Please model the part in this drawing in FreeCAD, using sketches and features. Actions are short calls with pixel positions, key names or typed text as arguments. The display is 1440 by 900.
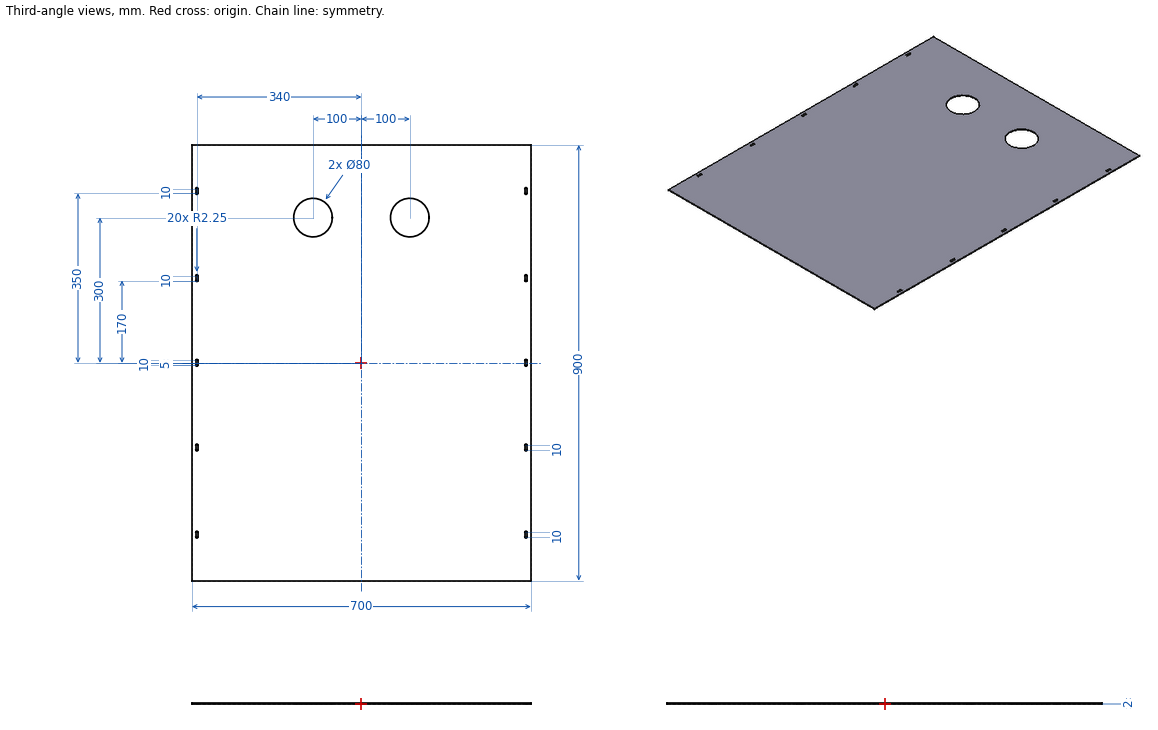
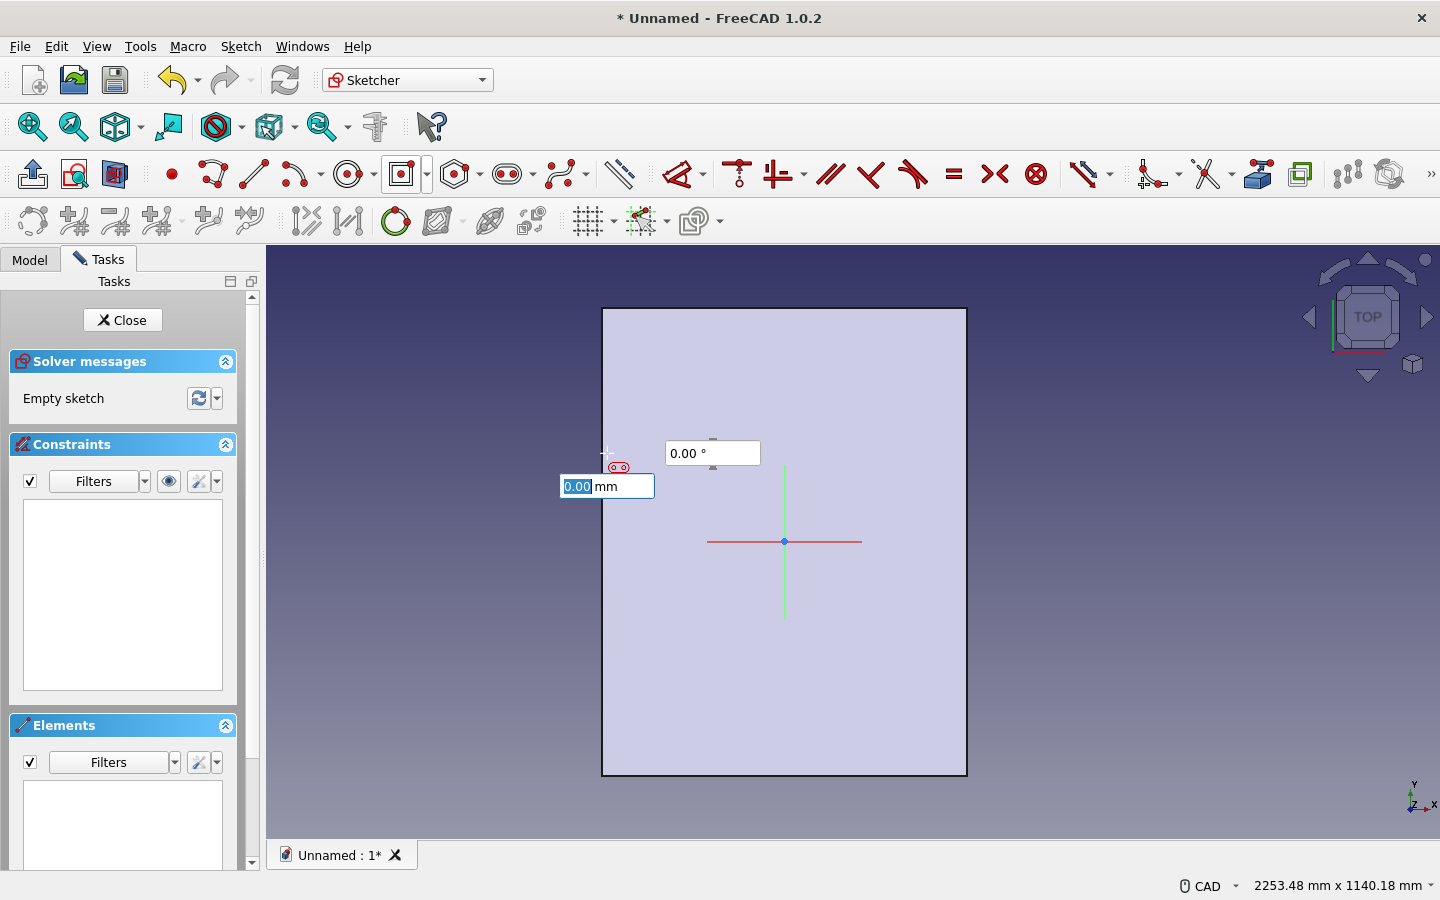
scroll(607, 448, up, 6)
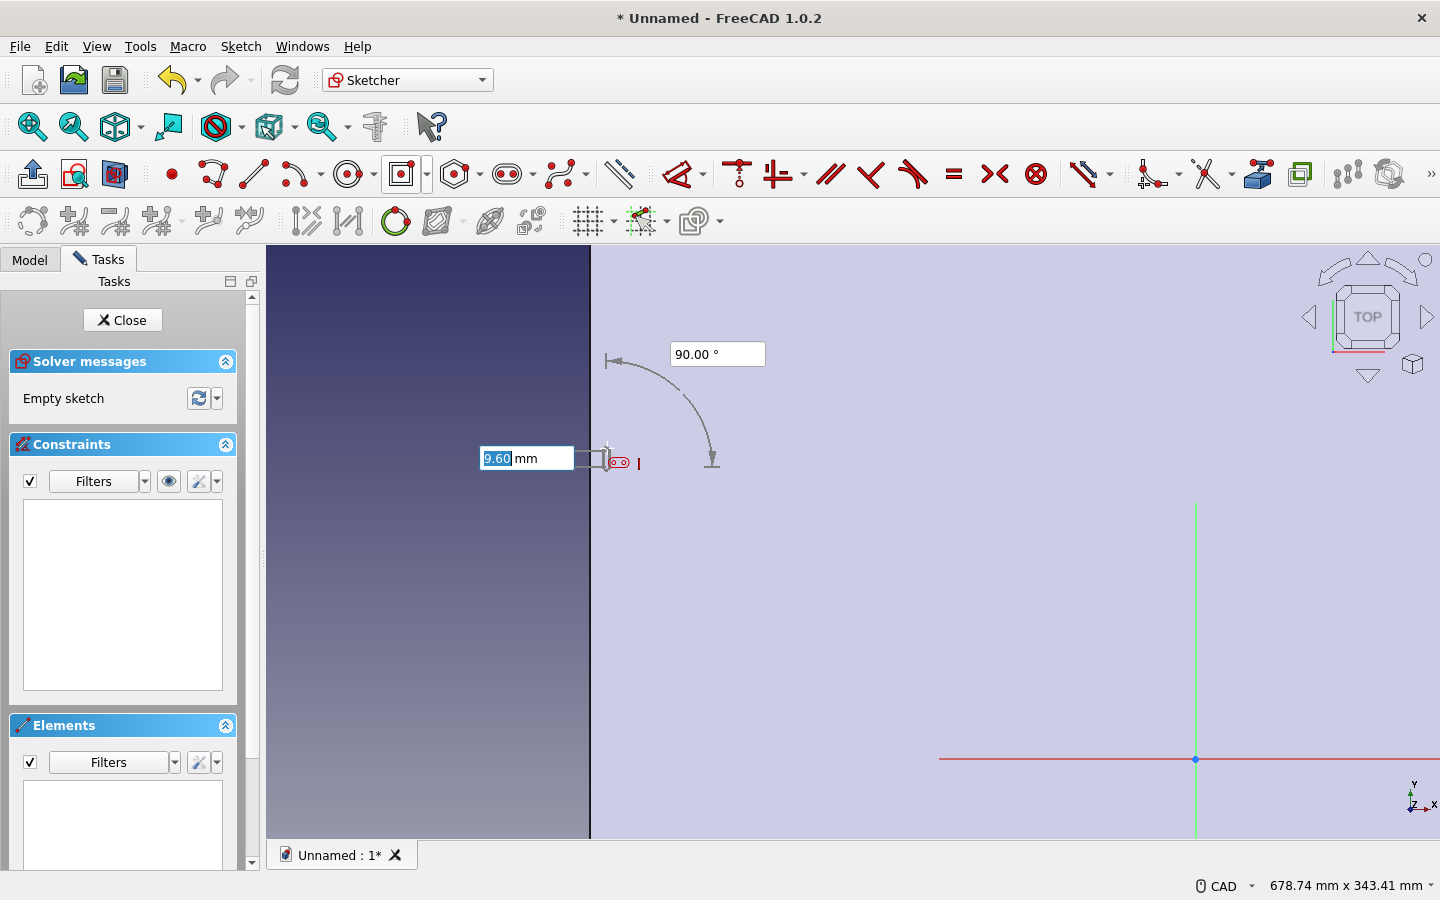
click(606, 448)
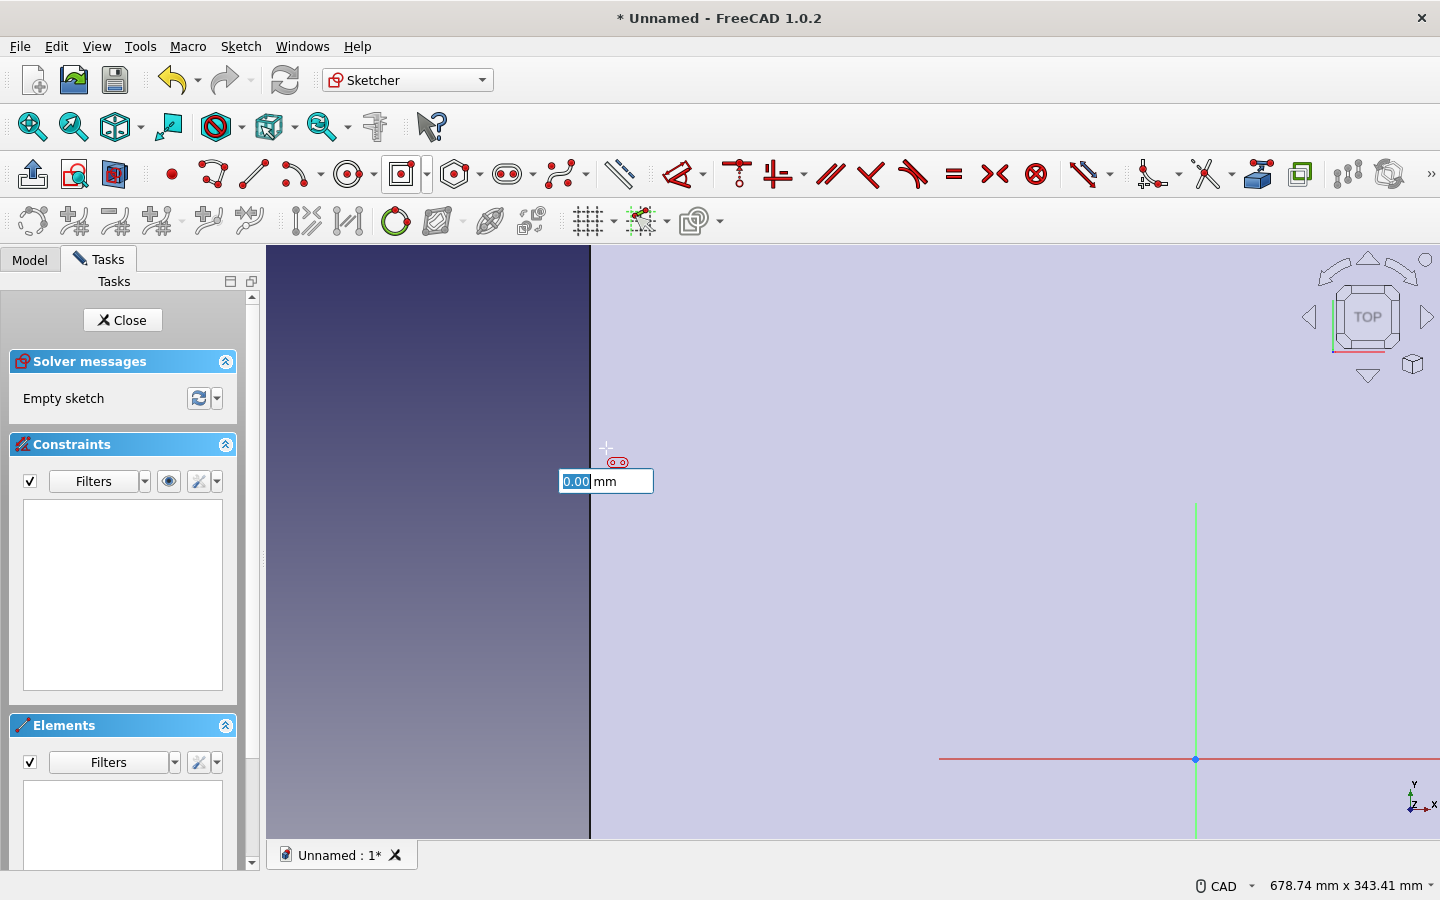
scroll(612, 457, up, 8)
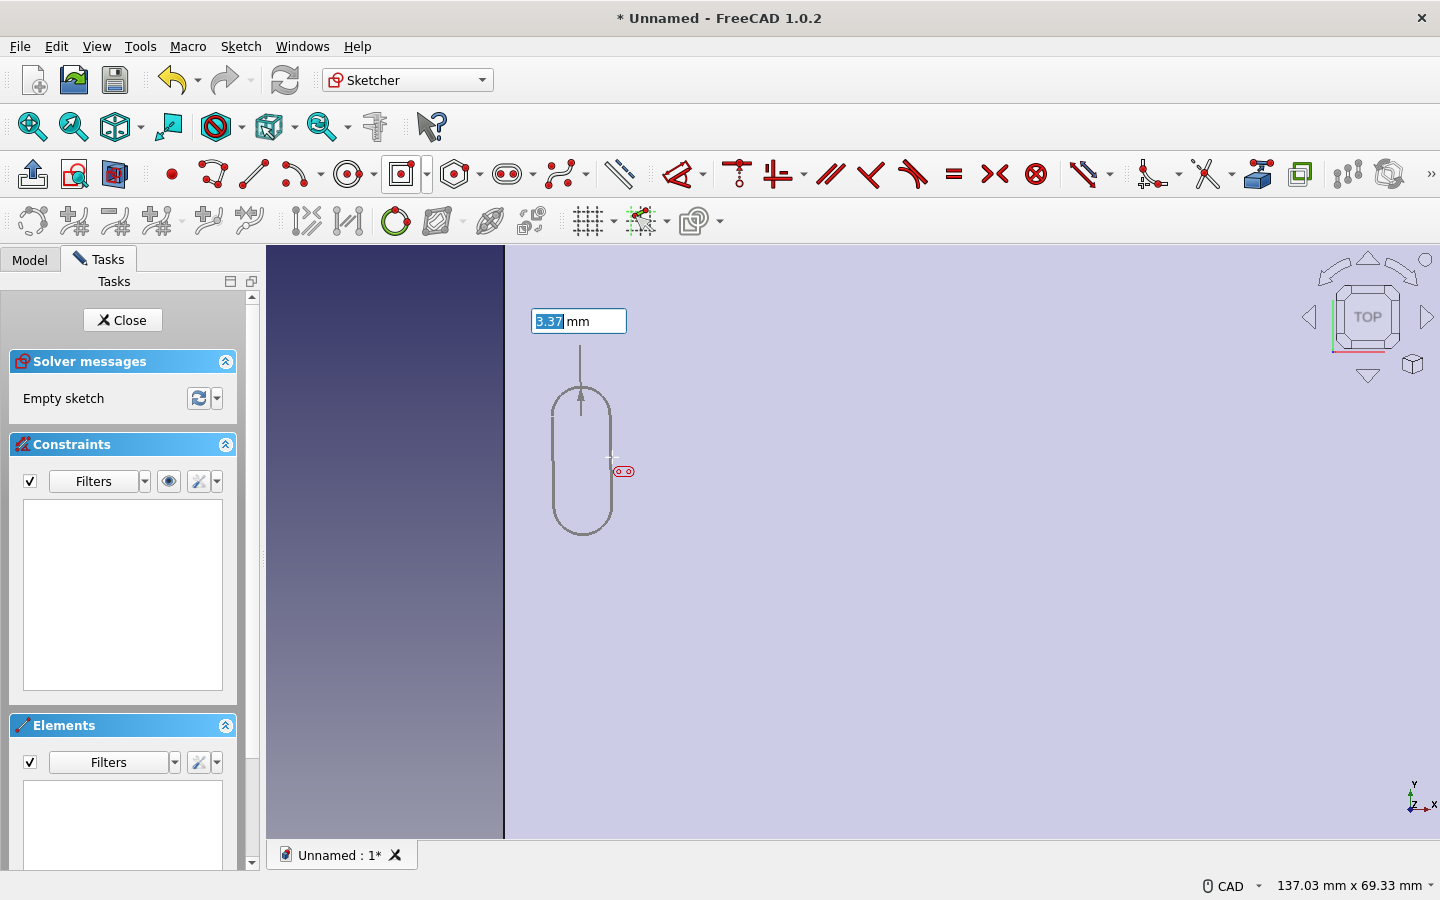
click(609, 454)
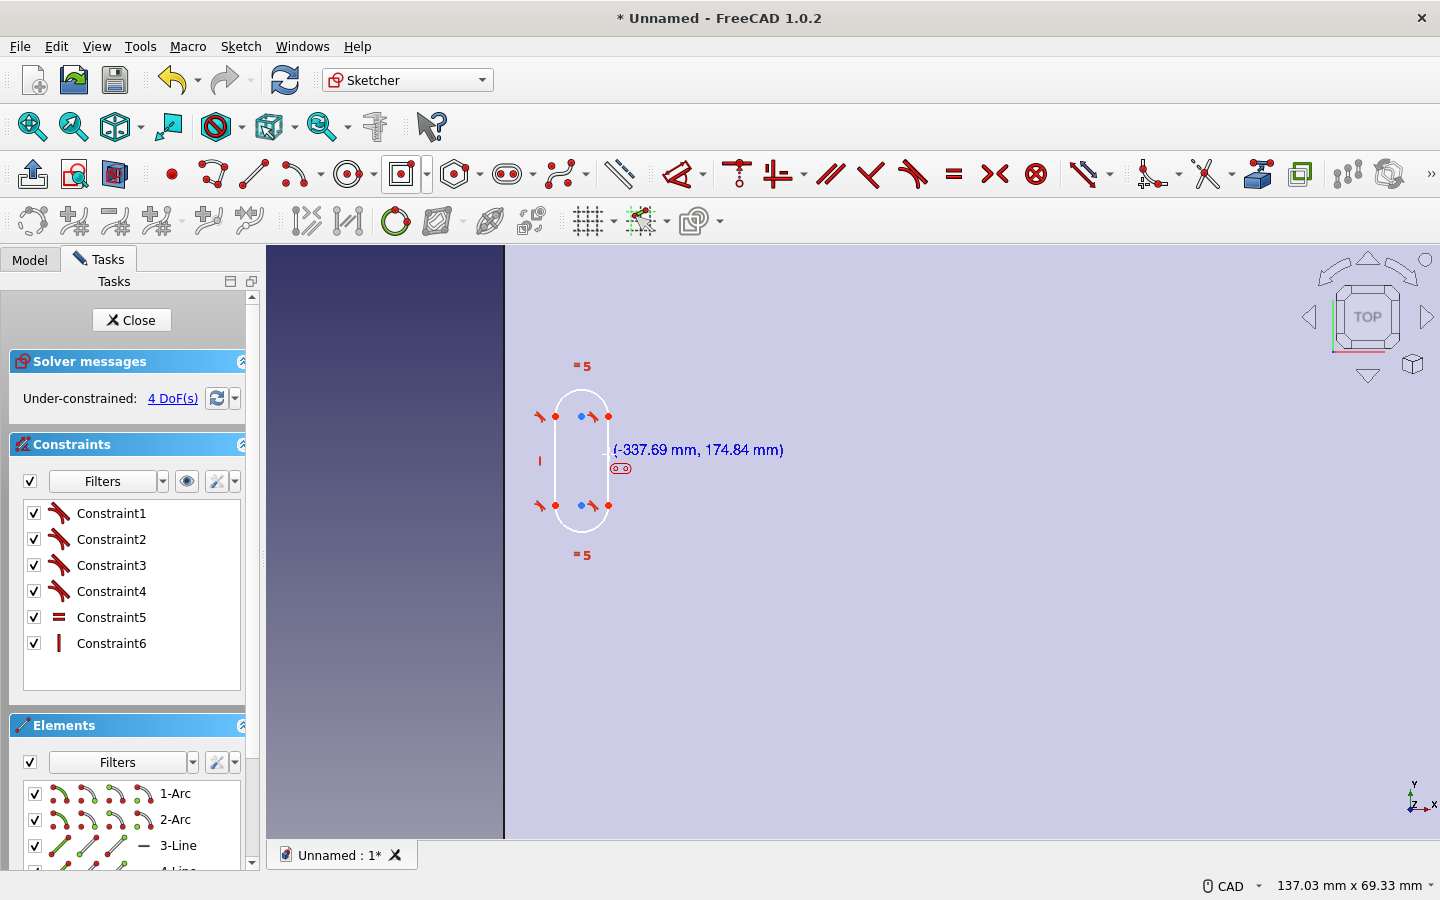
scroll(609, 451, down, 14)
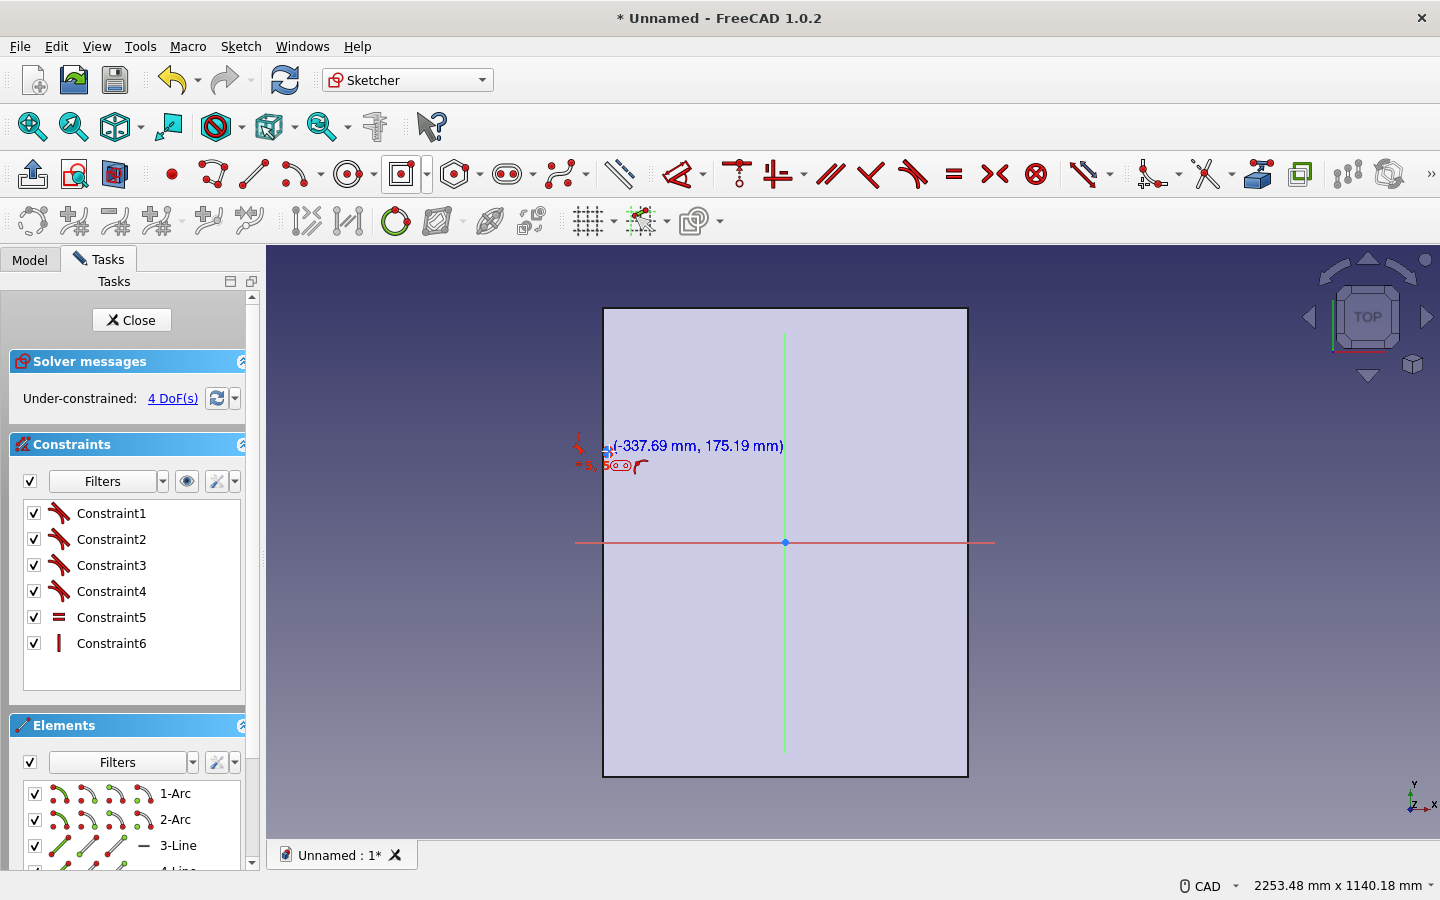
scroll(608, 545, up, 15)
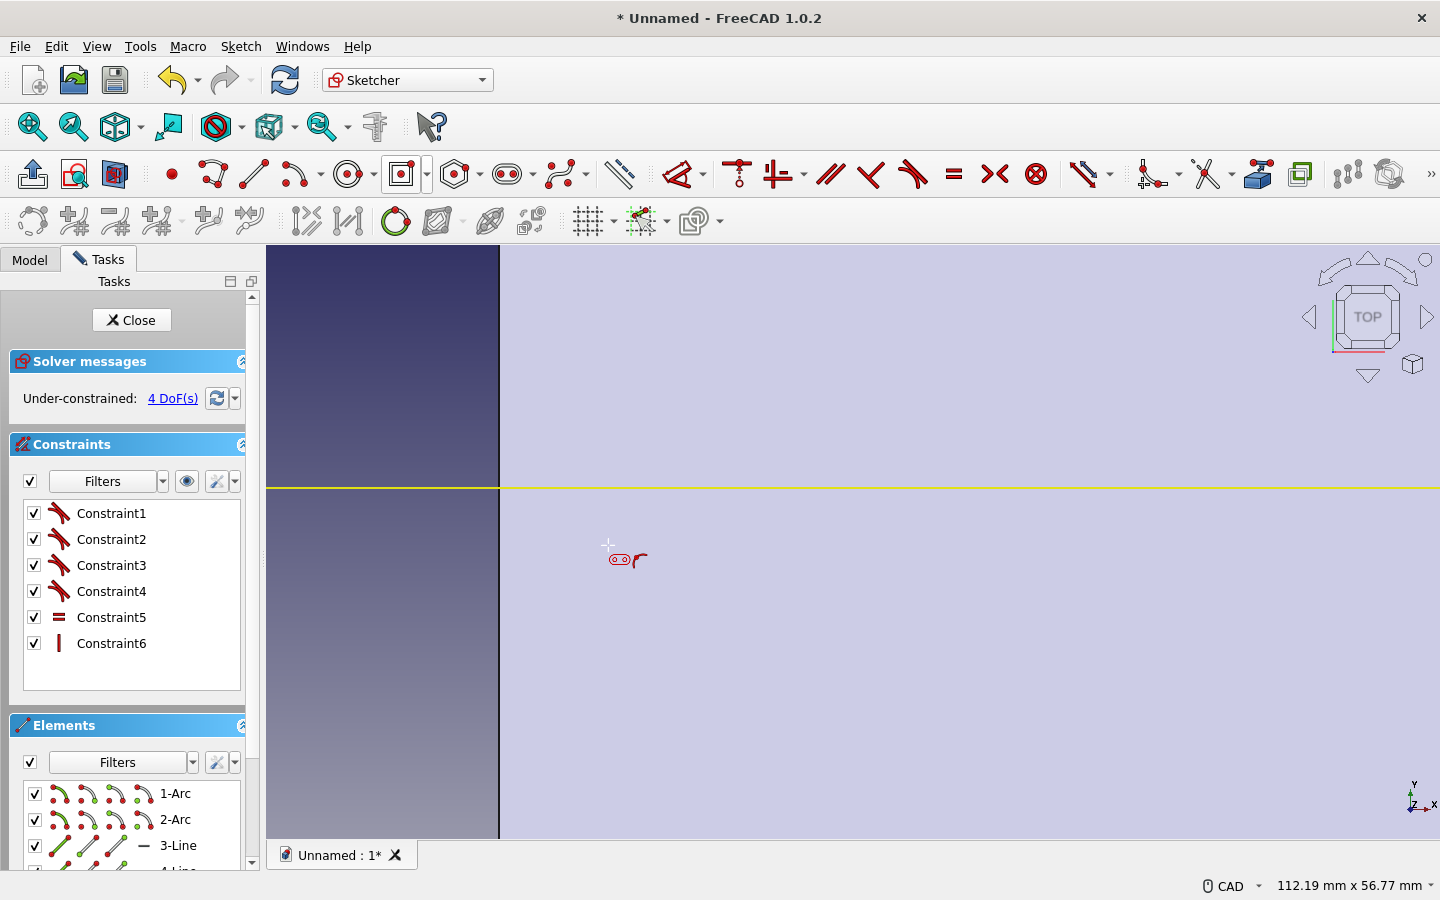
scroll(608, 545, down, 15)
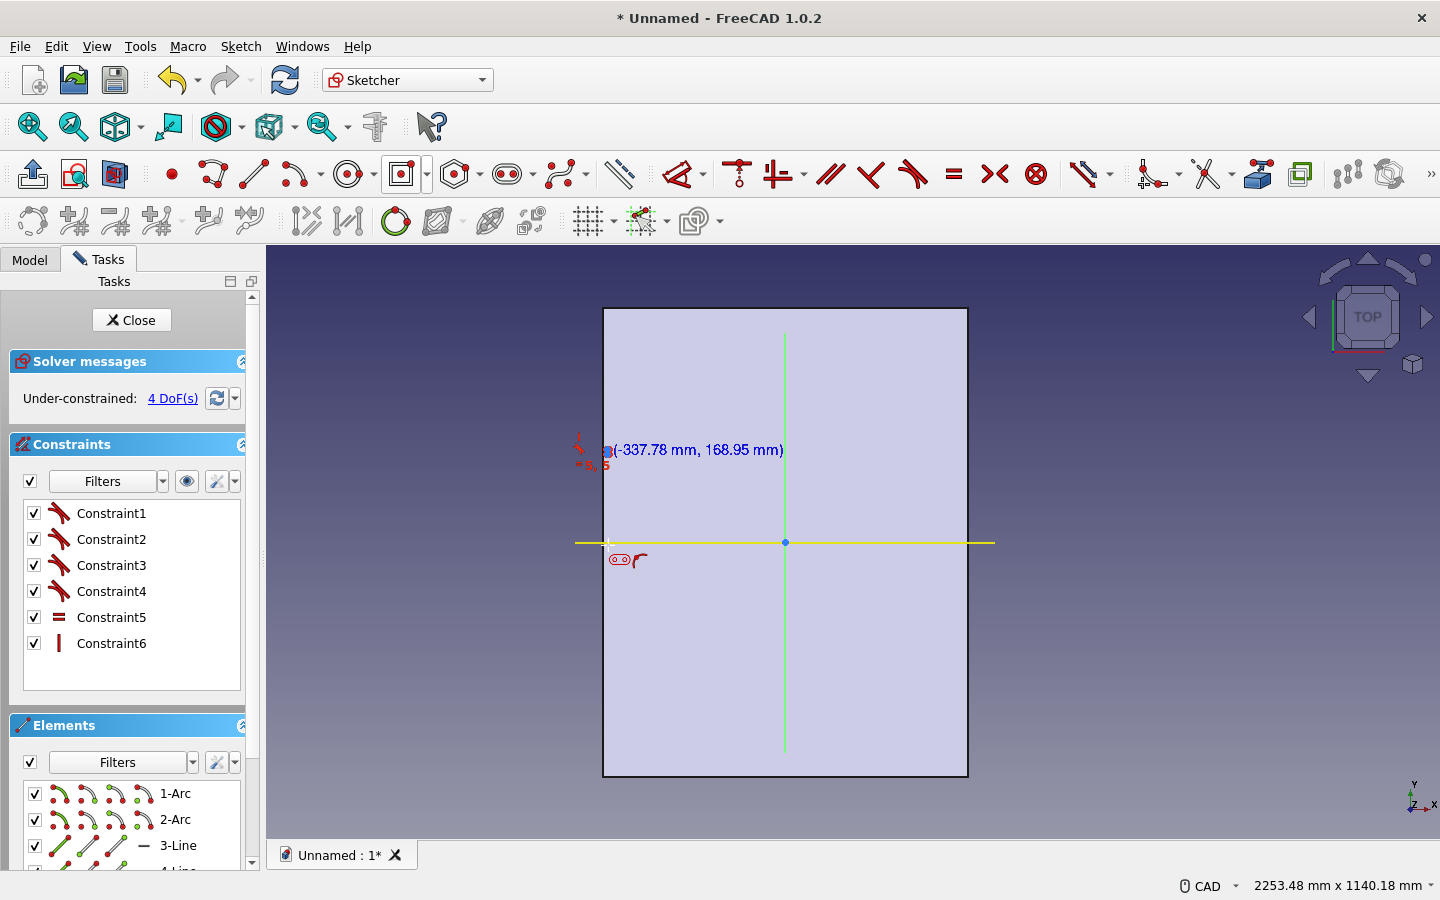
scroll(608, 545, up, 10)